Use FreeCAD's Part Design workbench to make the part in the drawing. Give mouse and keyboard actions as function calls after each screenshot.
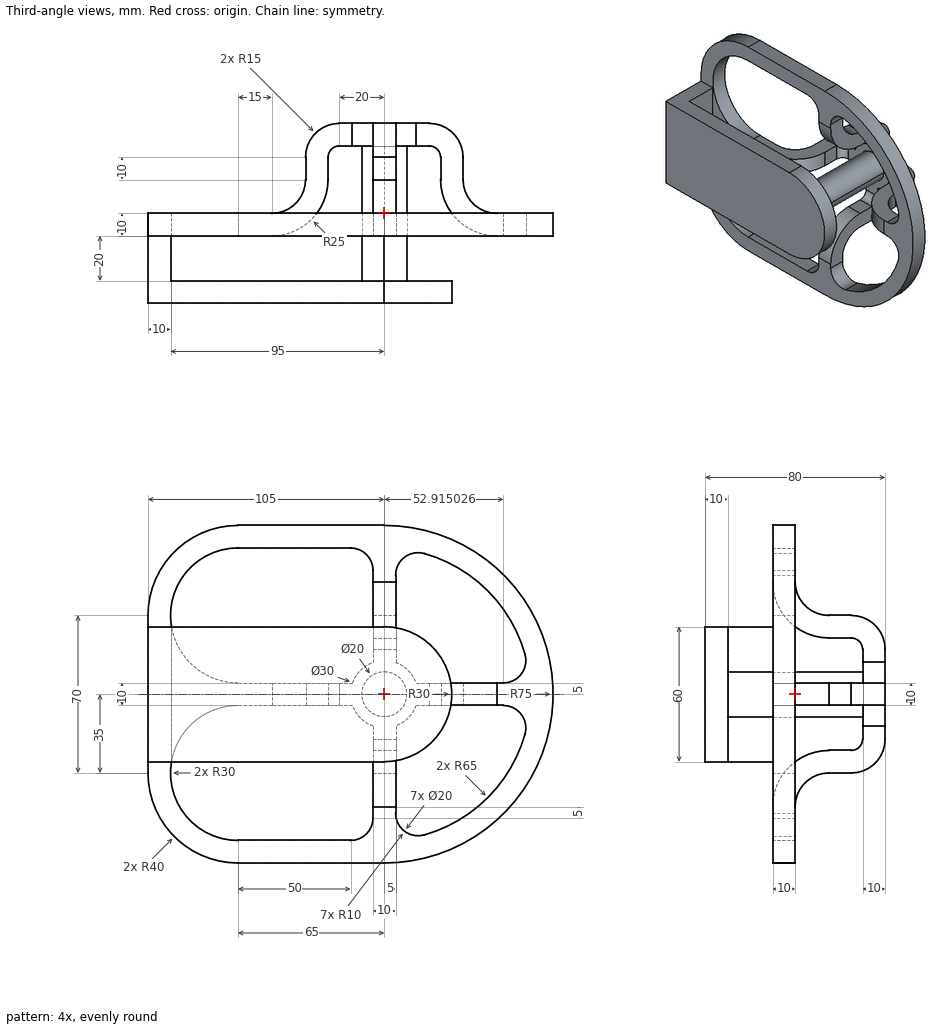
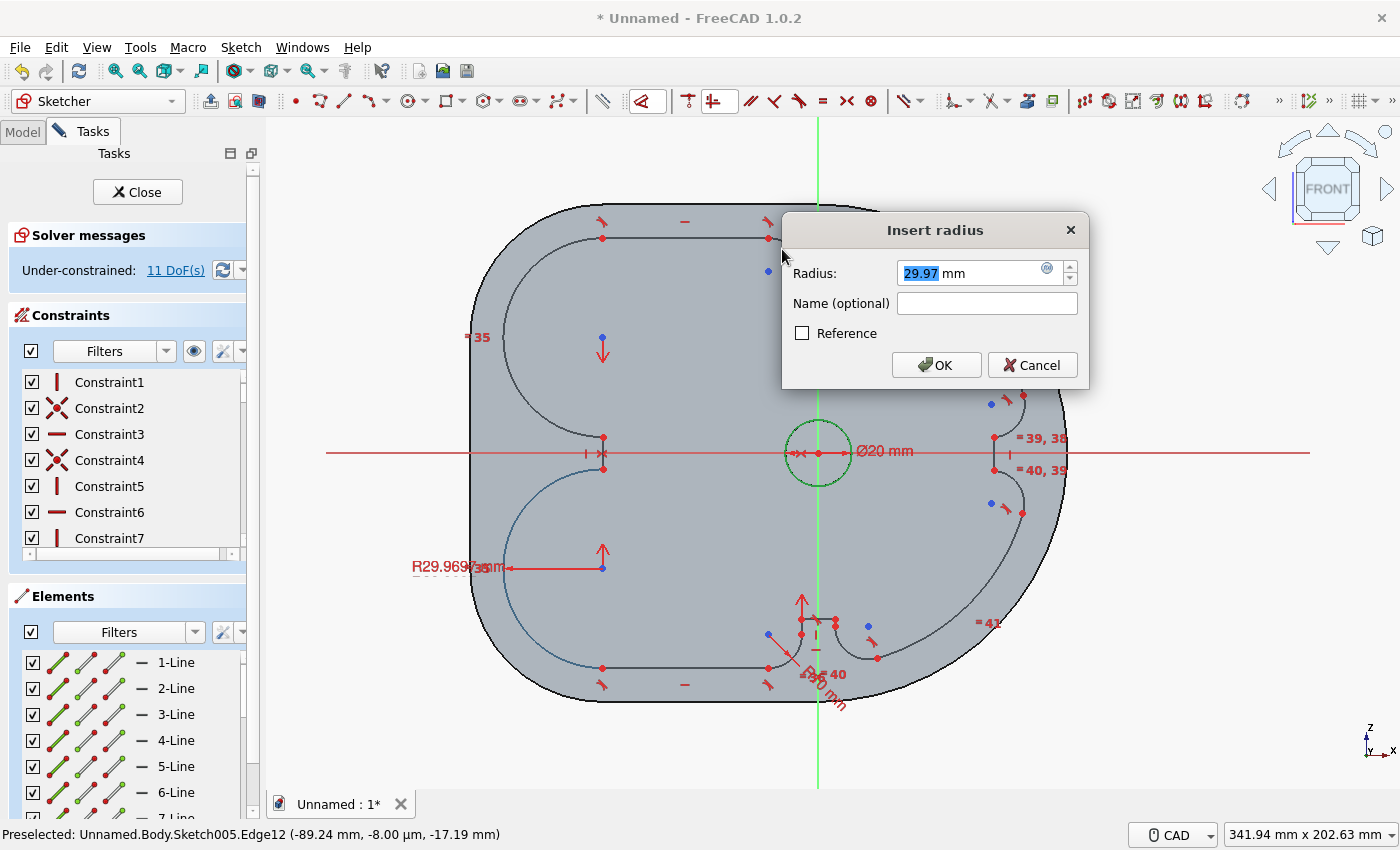
text(30)
key(Return)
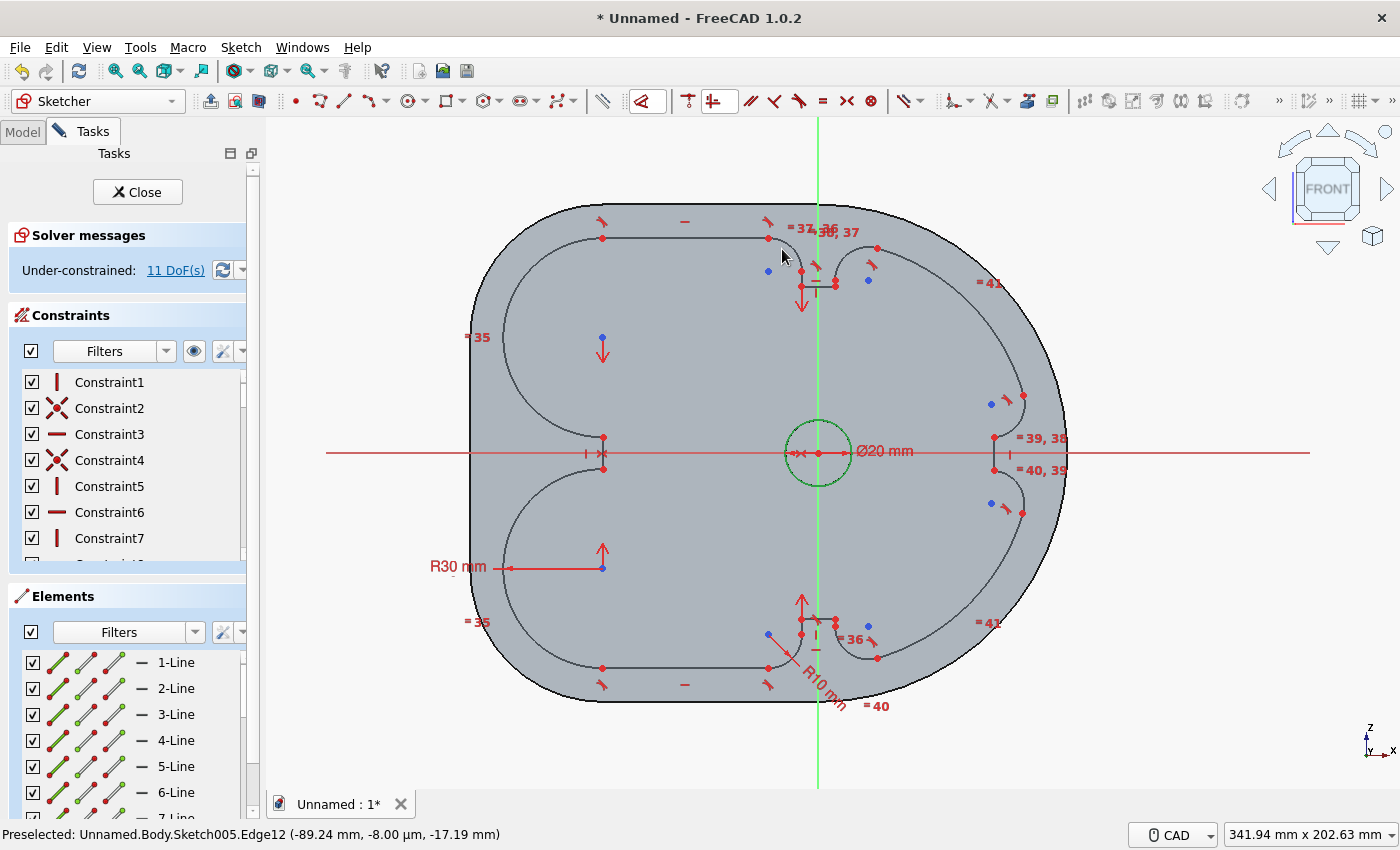
click(997, 336)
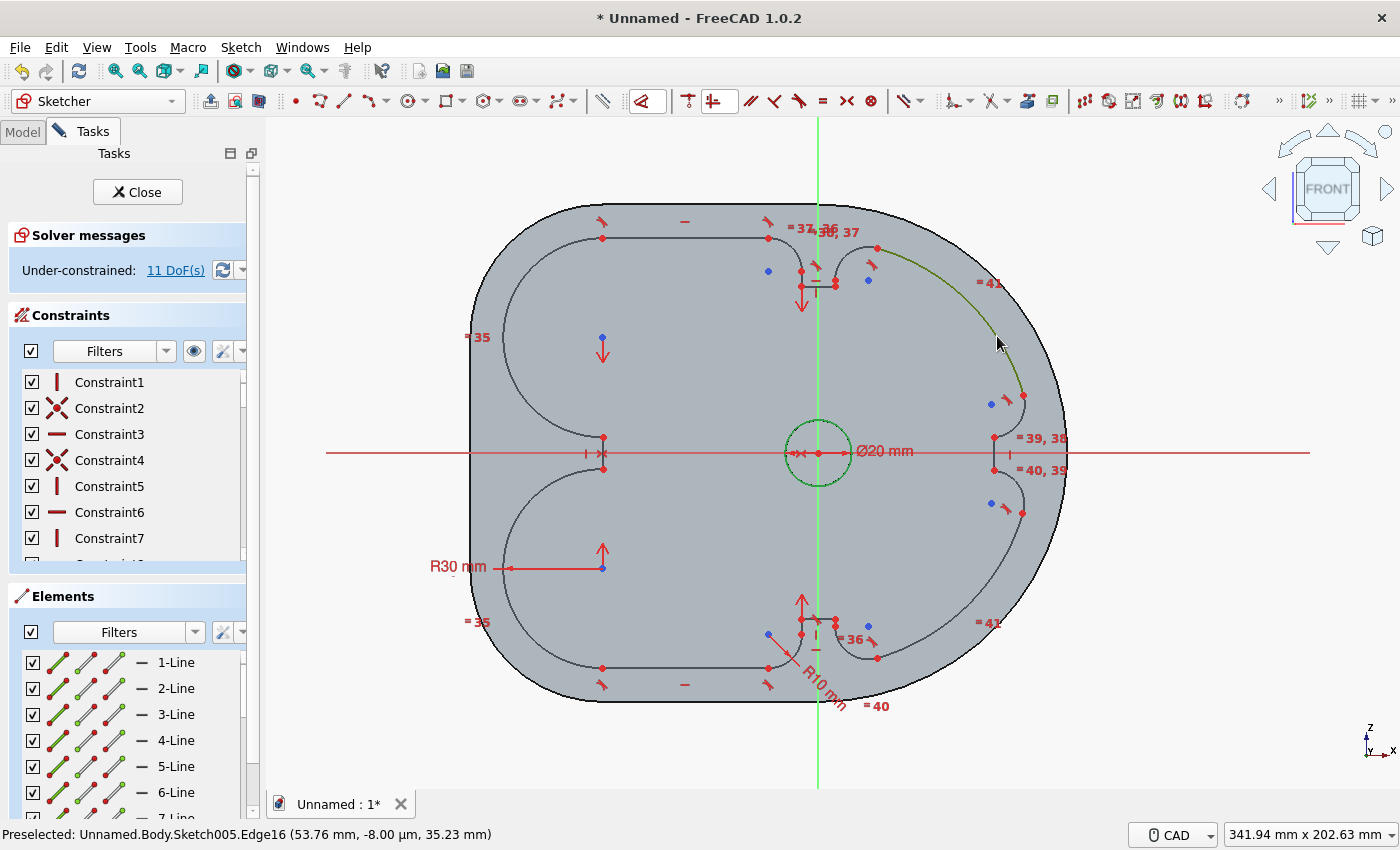
click(660, 102)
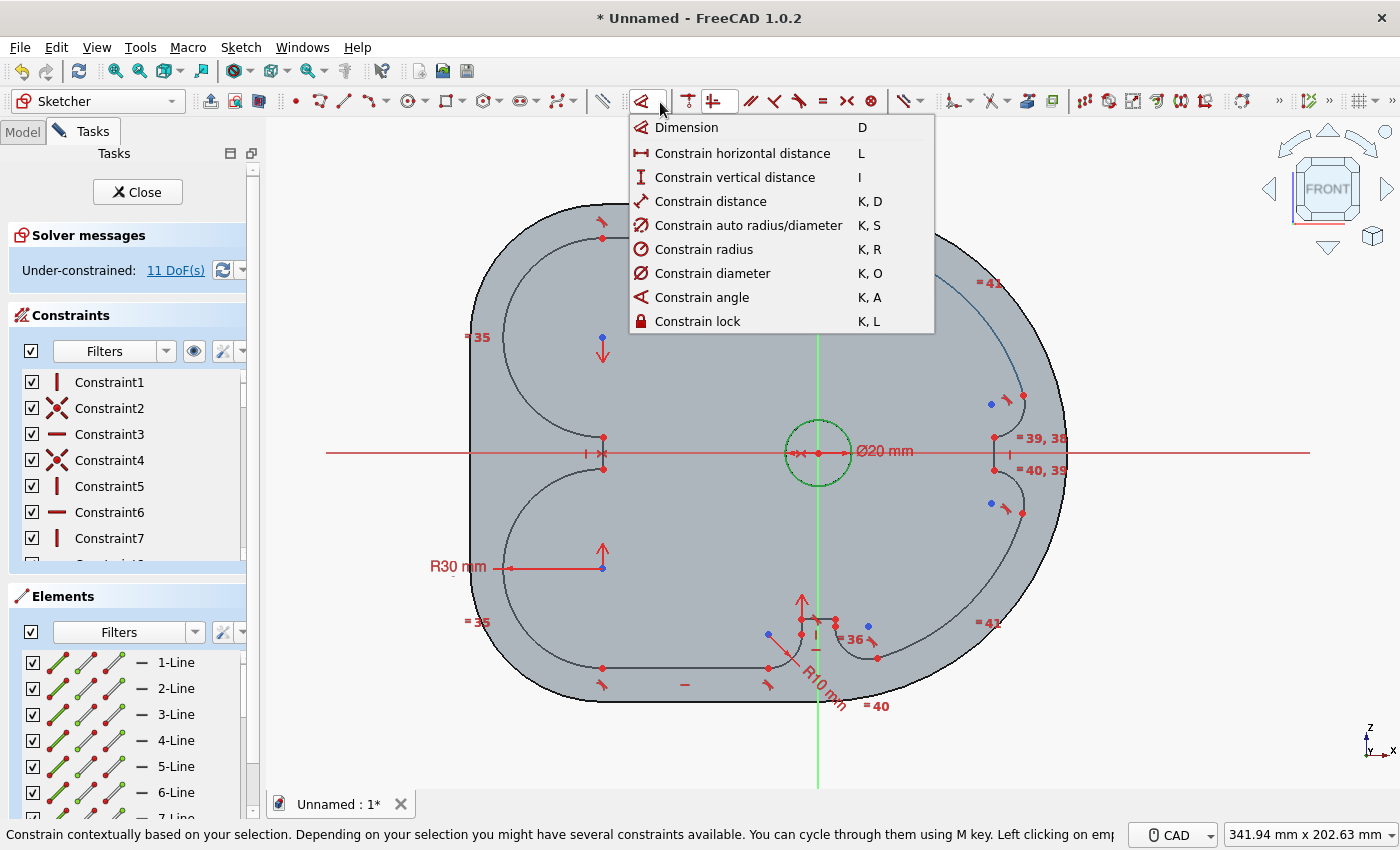
click(782, 249)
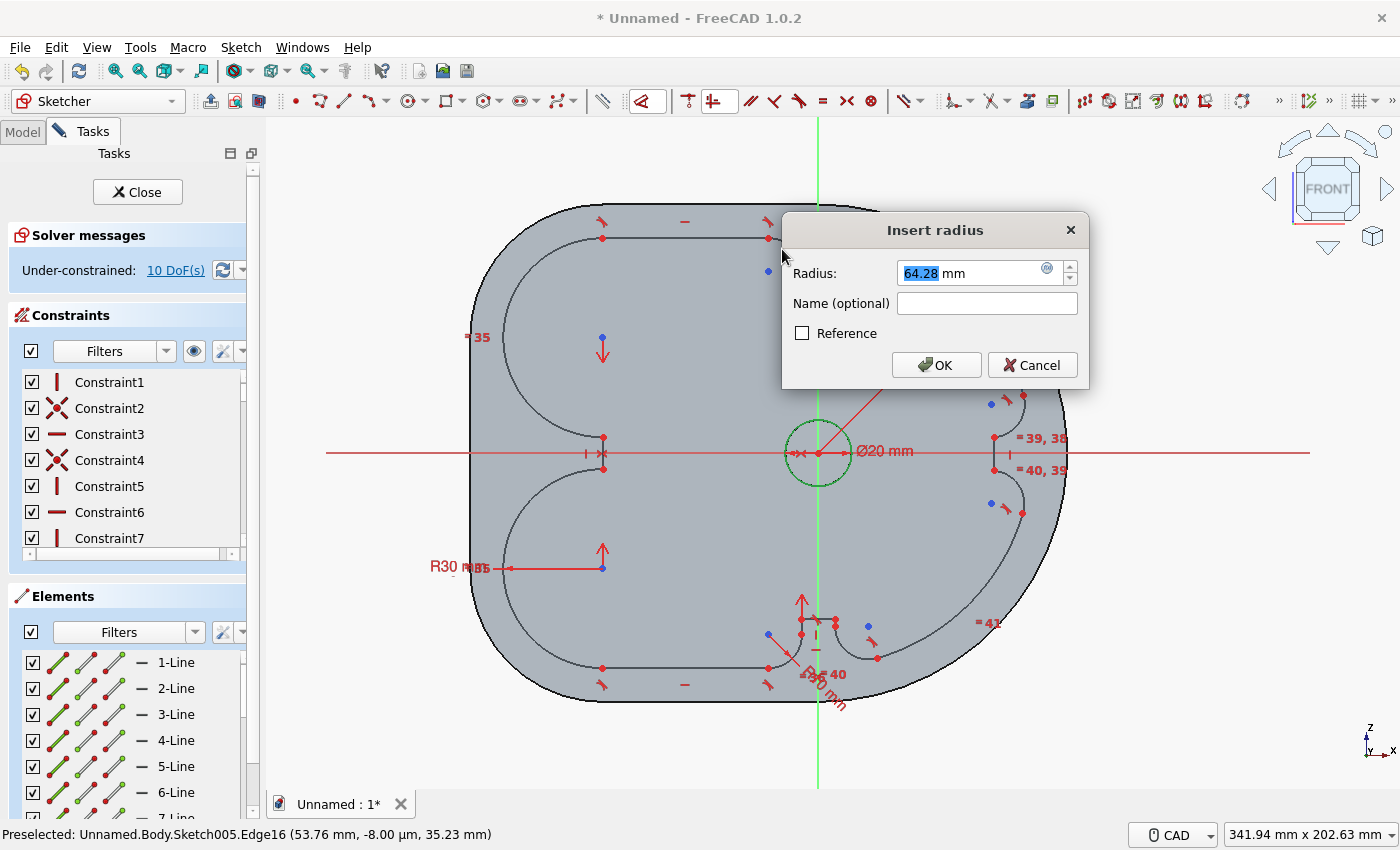
text(65)
key(Return)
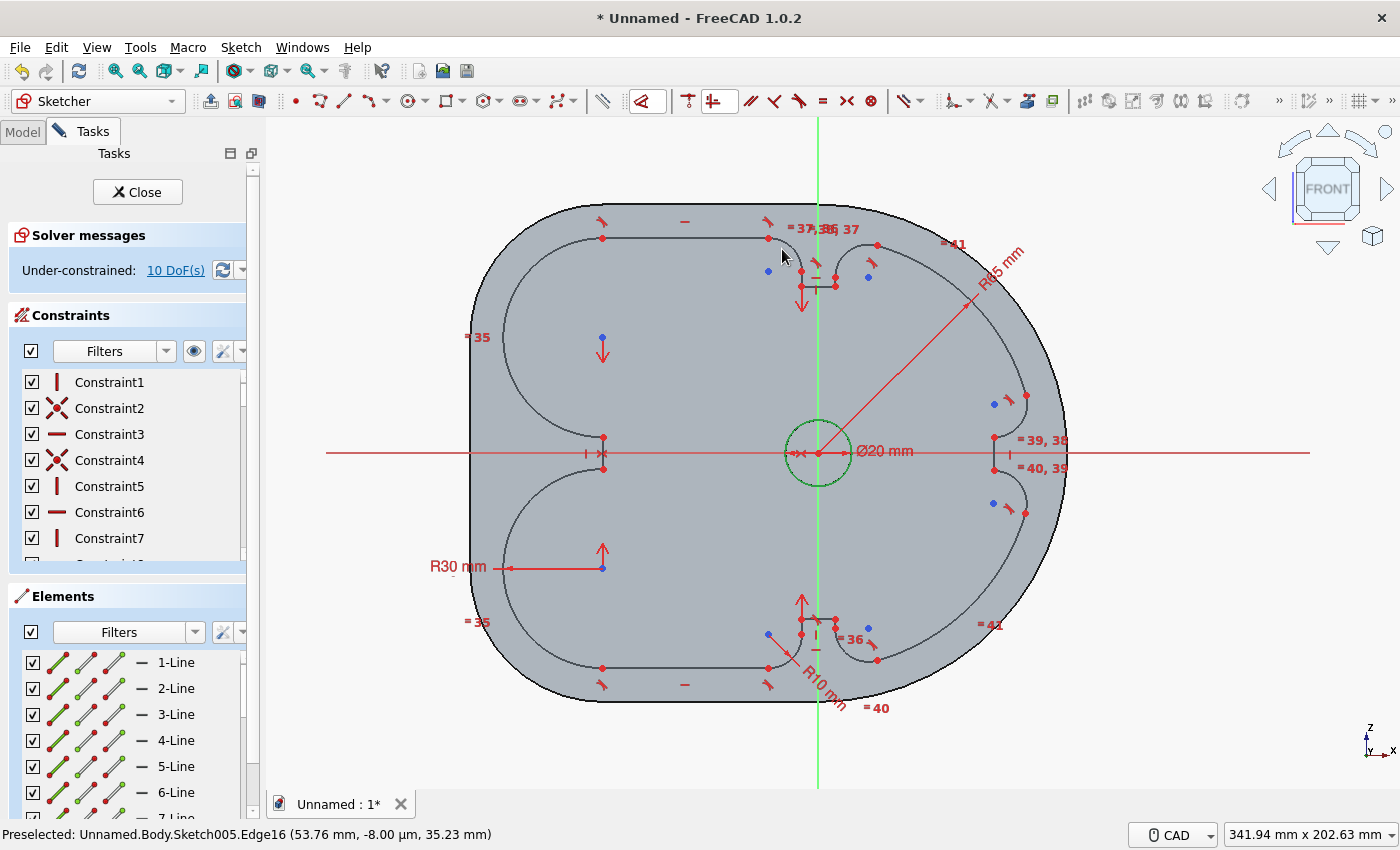
scroll(802, 627, up, 5)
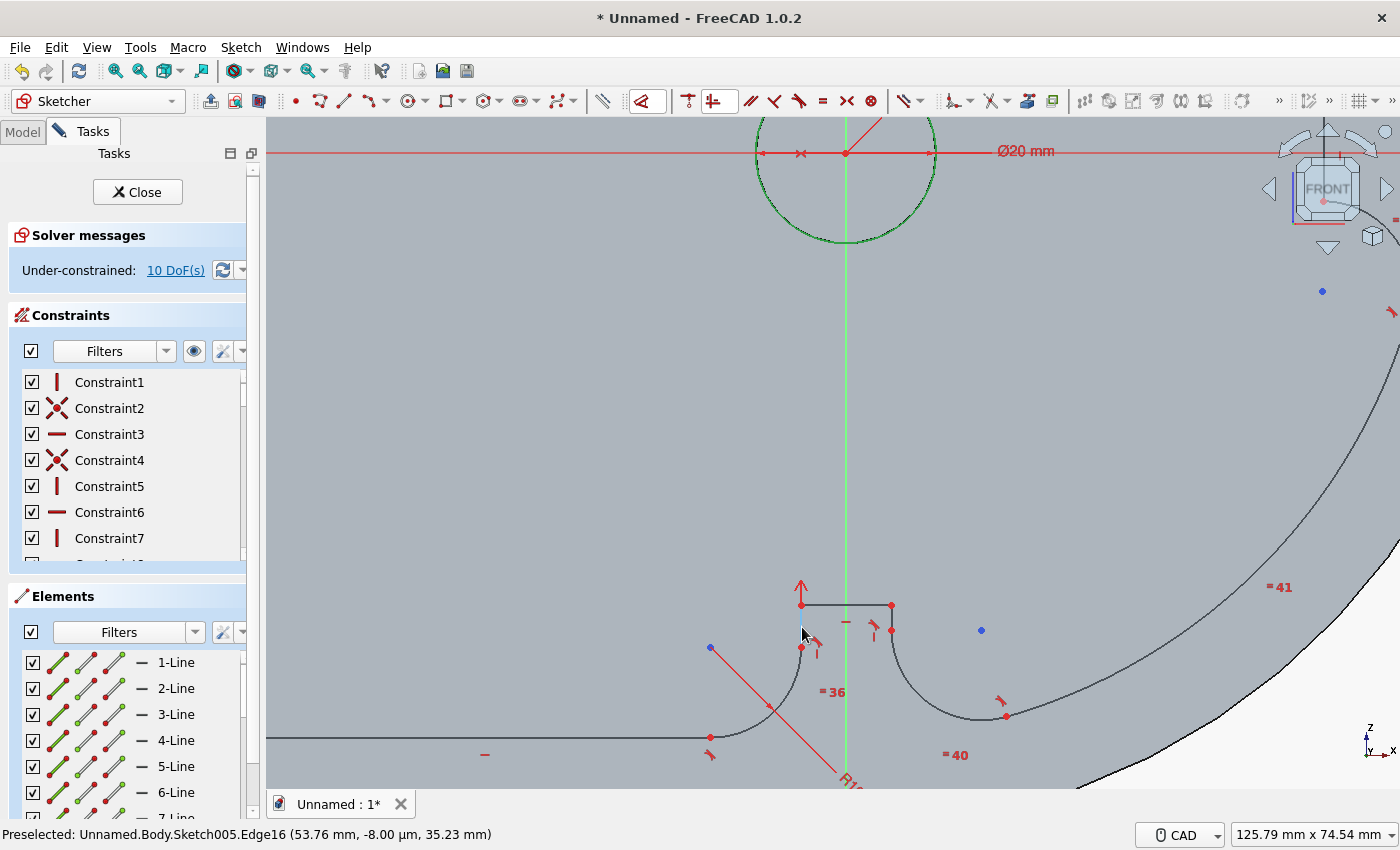
click(801, 626)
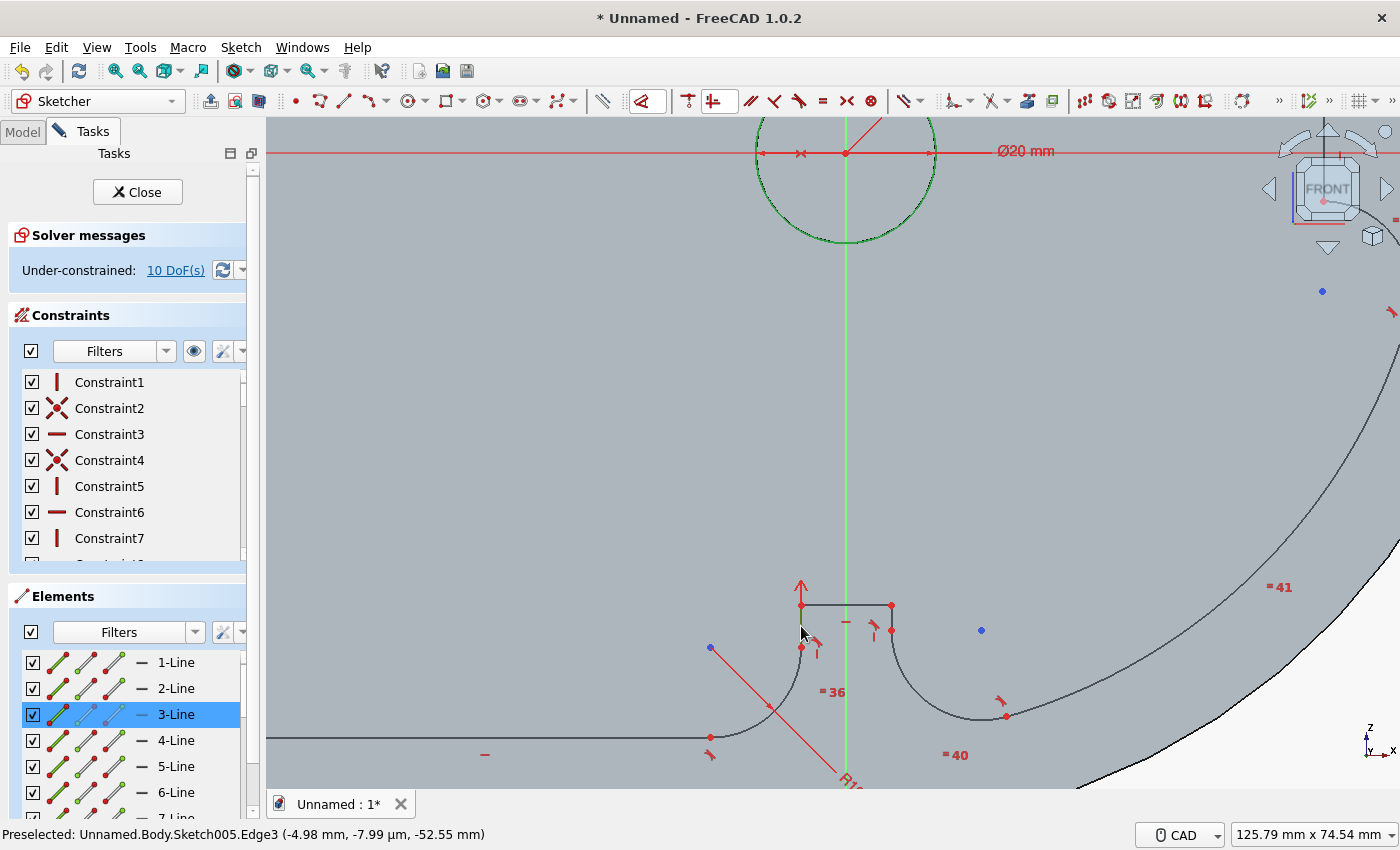
click(660, 102)